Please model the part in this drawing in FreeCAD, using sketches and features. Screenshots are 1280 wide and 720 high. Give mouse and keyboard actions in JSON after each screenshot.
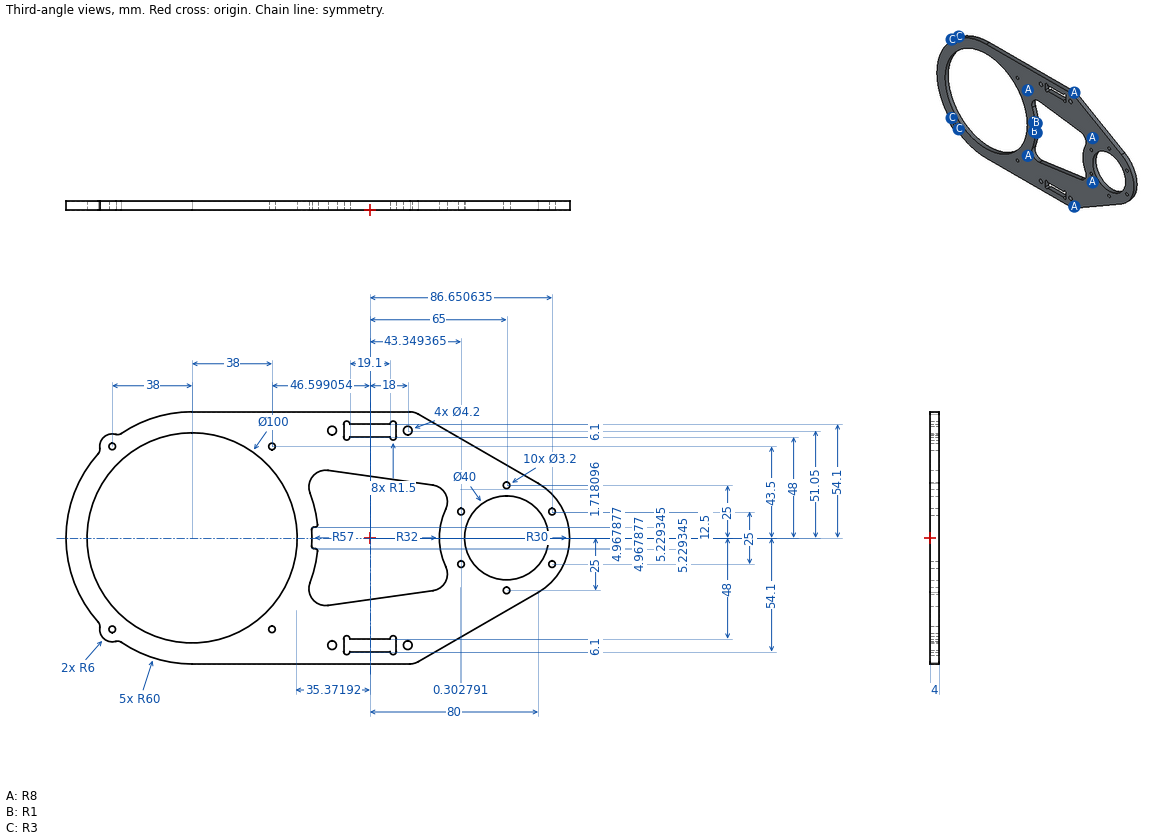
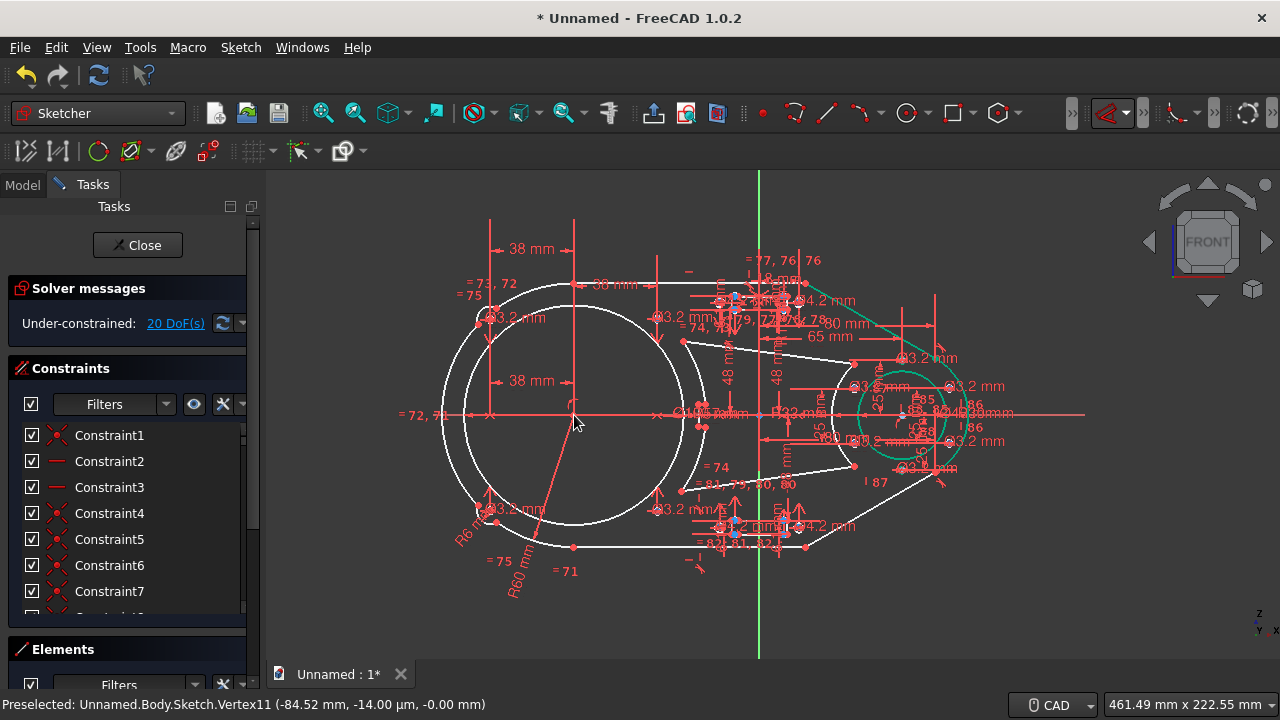
{"action": "left_click", "coordinate": [574, 547]}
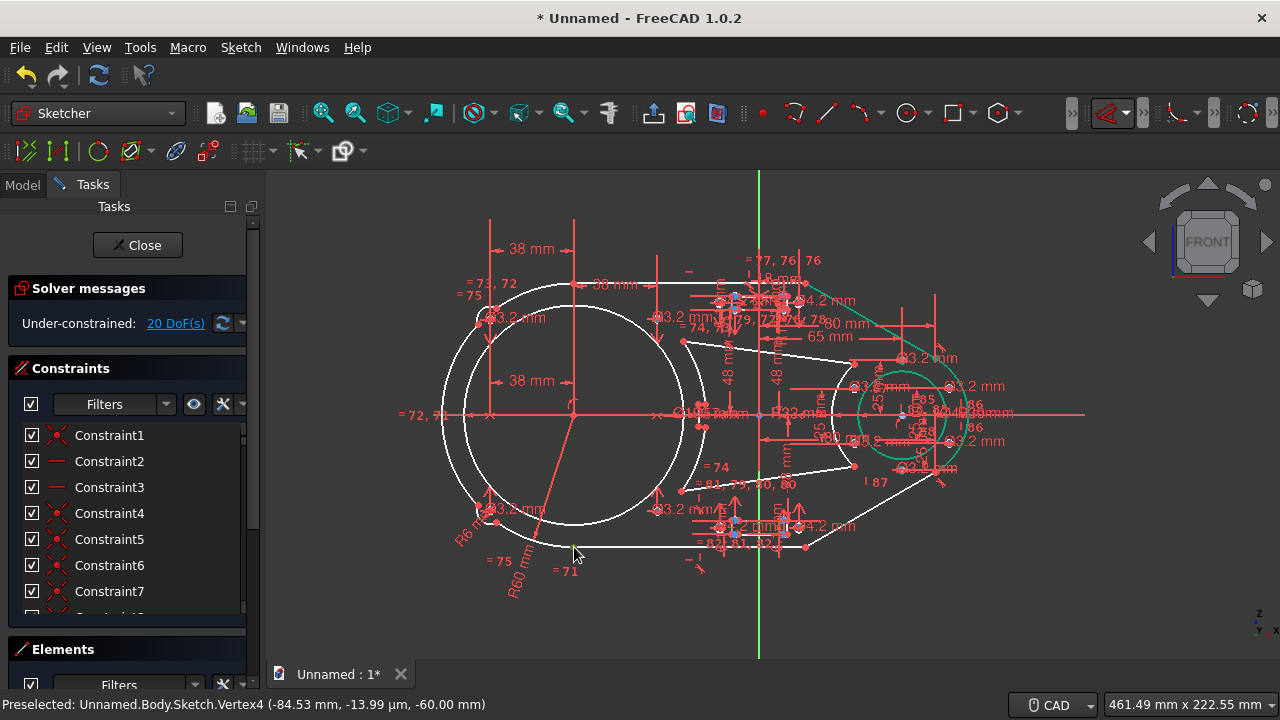
{"action": "left_click", "coordinate": [490, 511]}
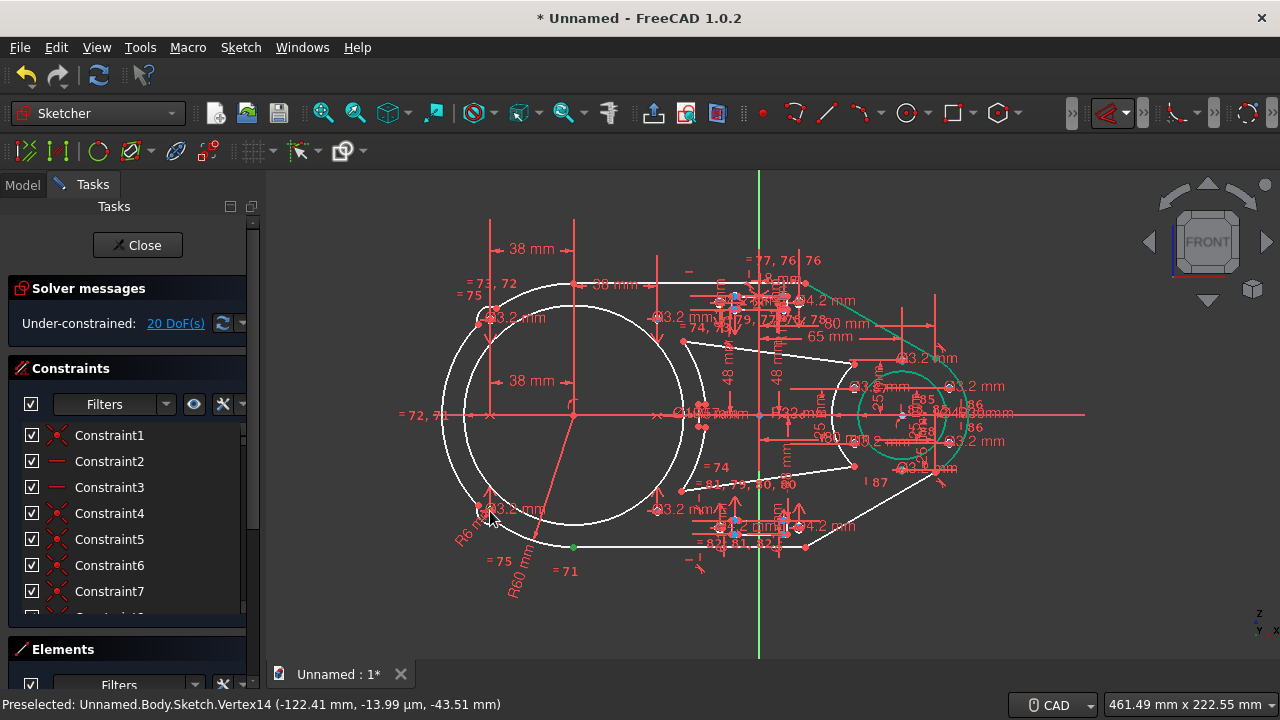
{"action": "left_click", "coordinate": [1128, 114]}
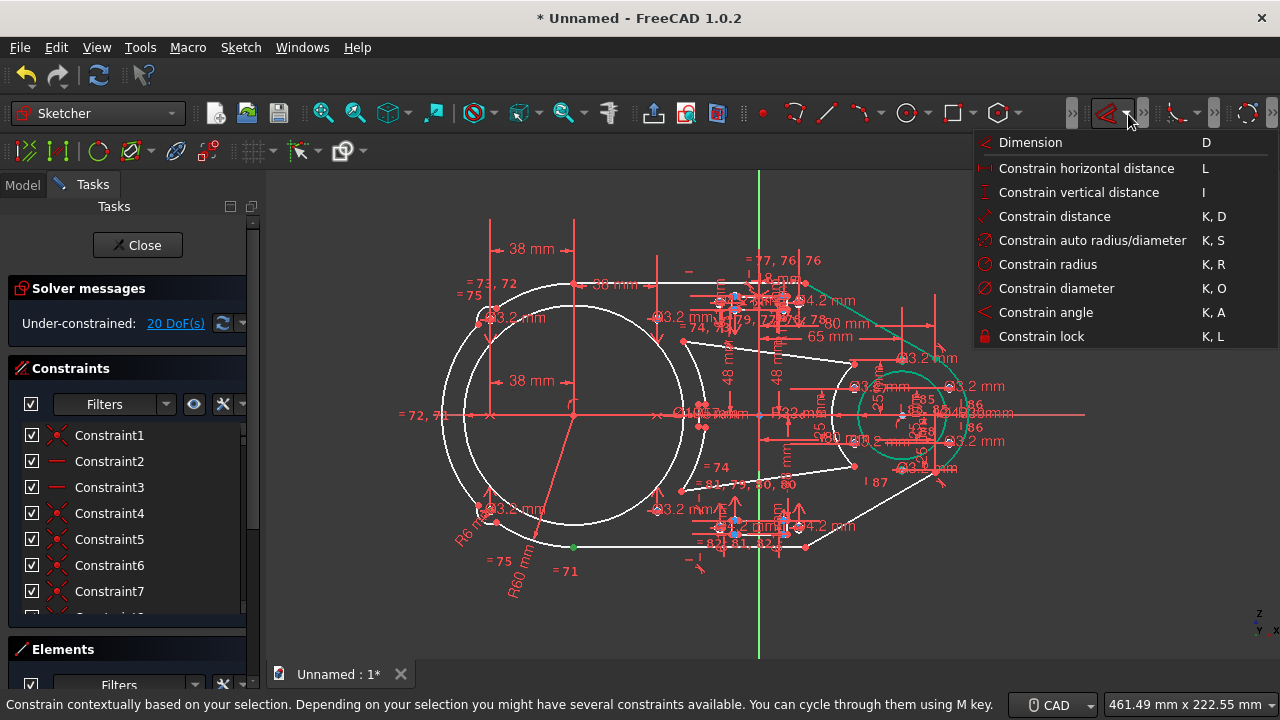
{"action": "left_click", "coordinate": [1126, 168]}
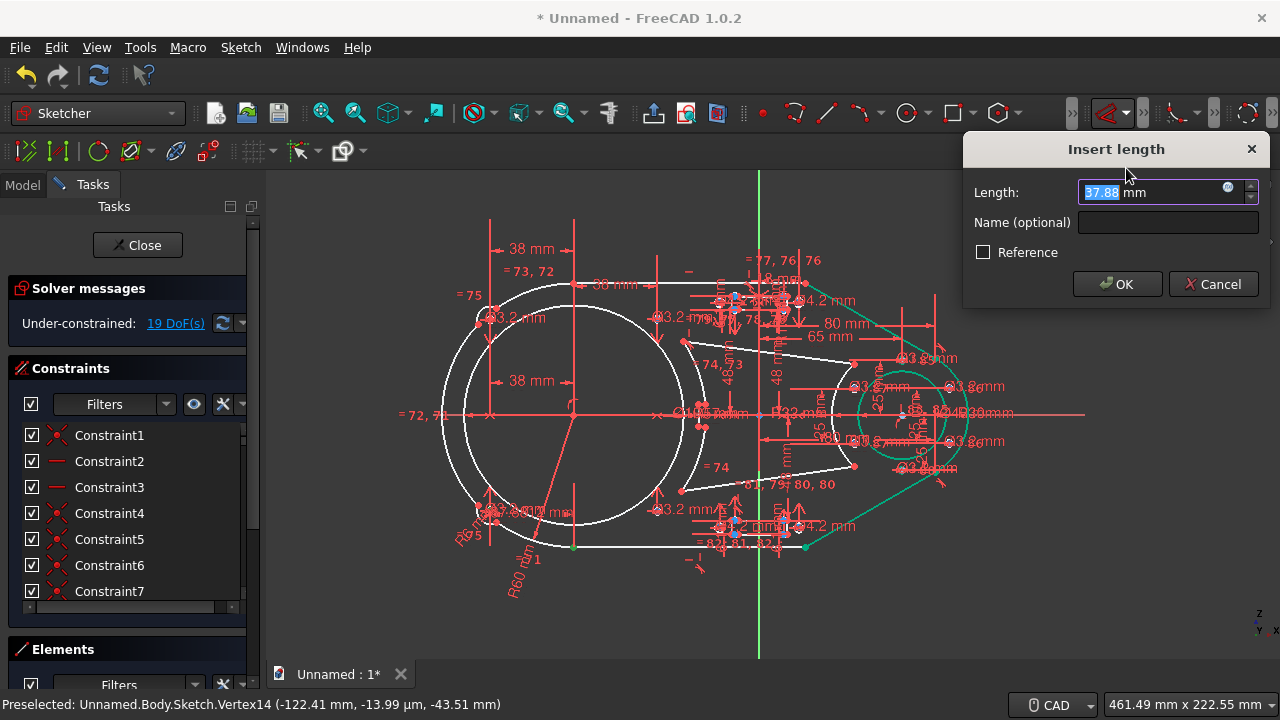
{"action": "type", "text": "38"}
{"action": "key", "text": "Return"}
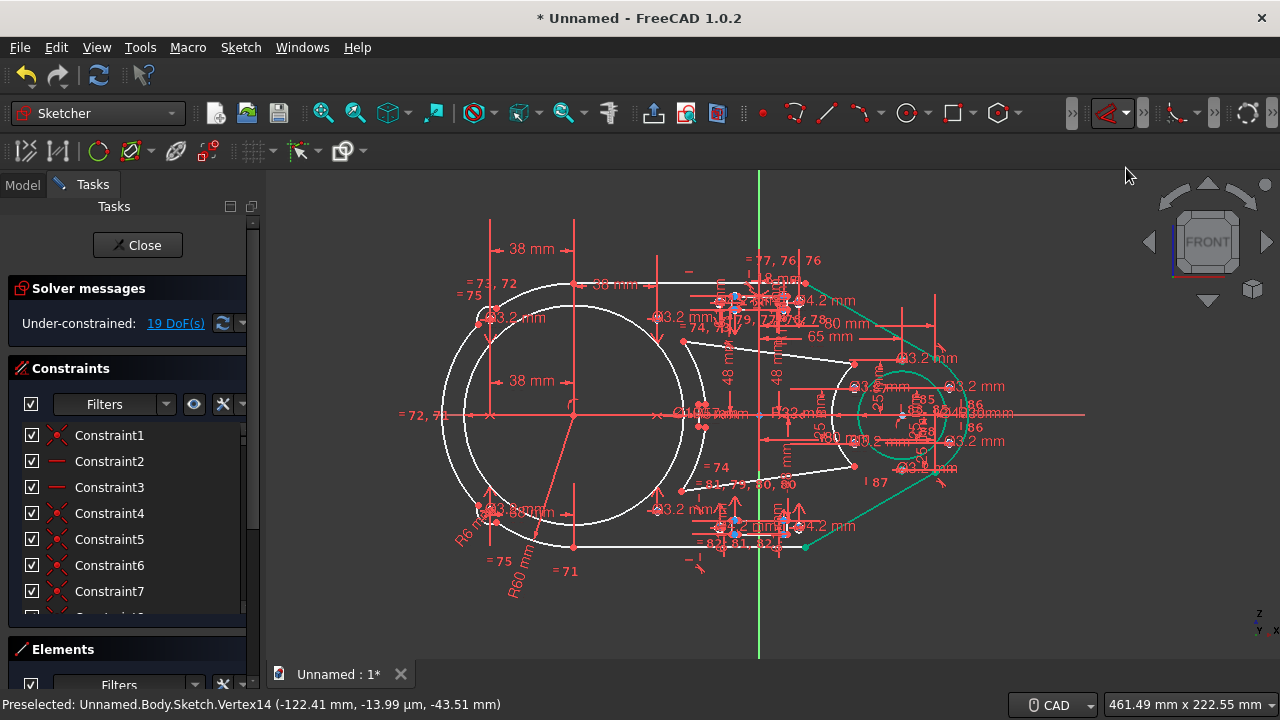
{"action": "left_click", "coordinate": [747, 310]}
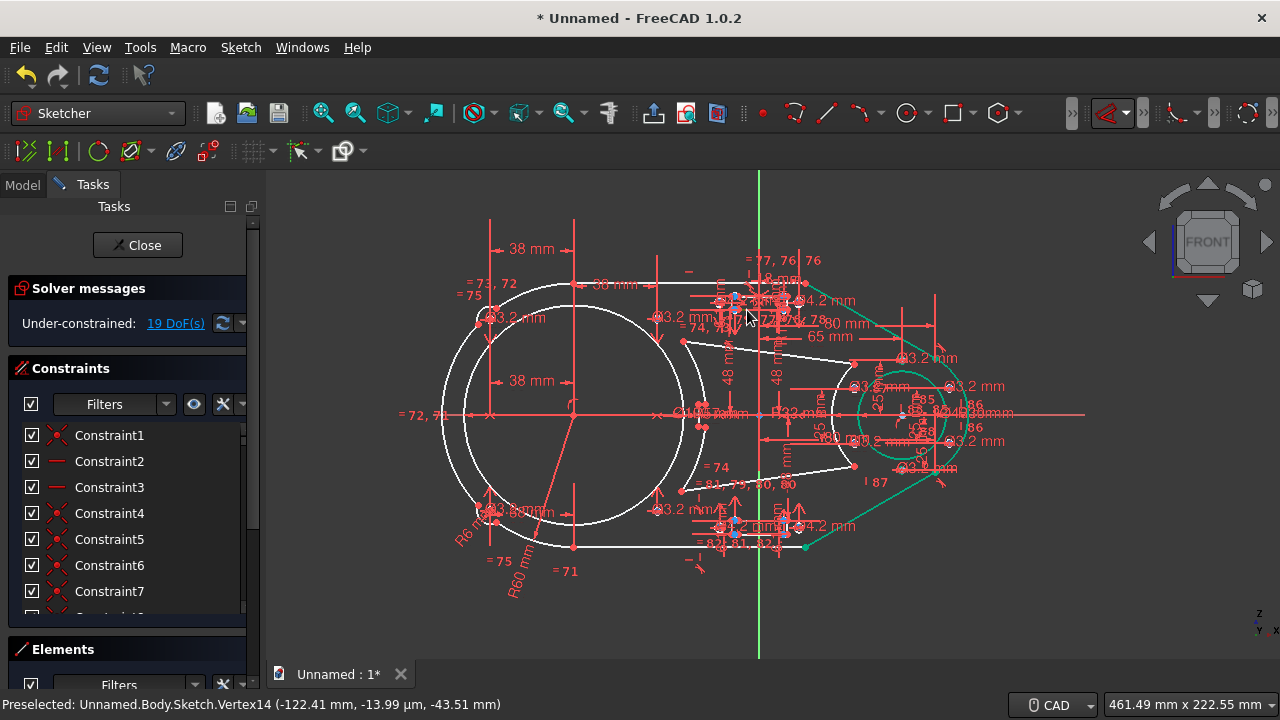
{"action": "key", "text": "l"}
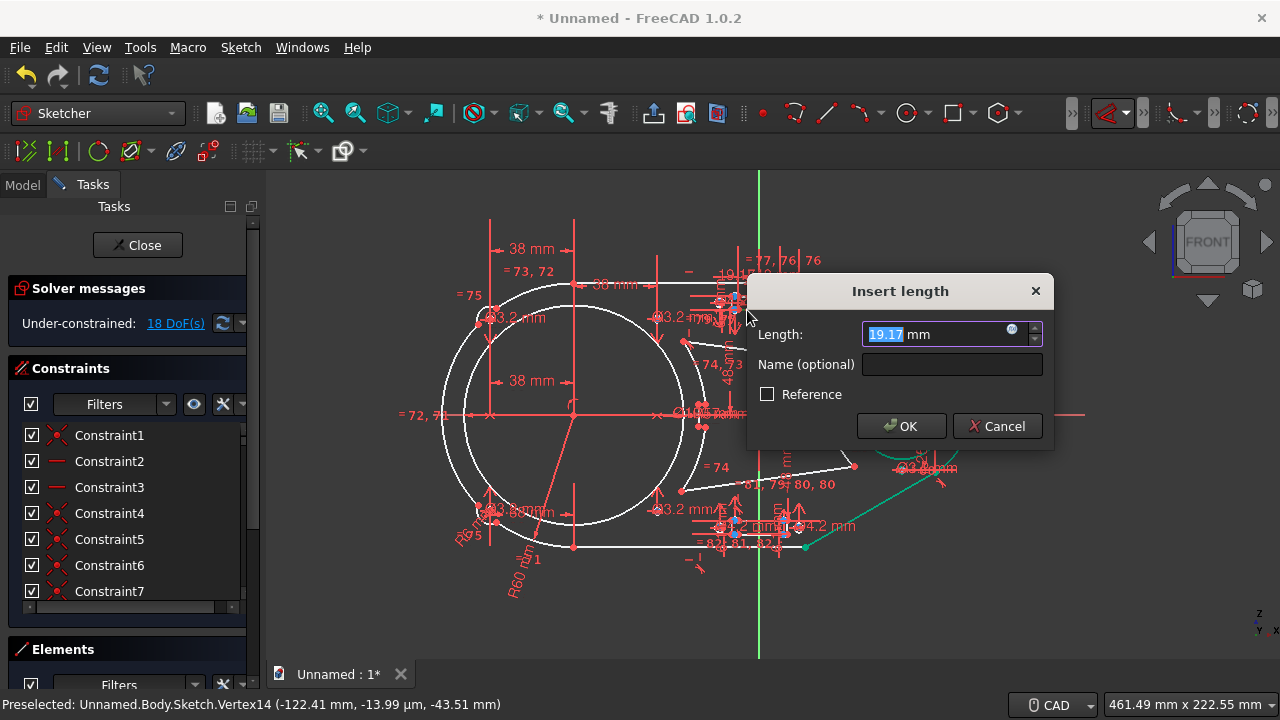
{"action": "type", "text": "19.1"}
{"action": "key", "text": "Return"}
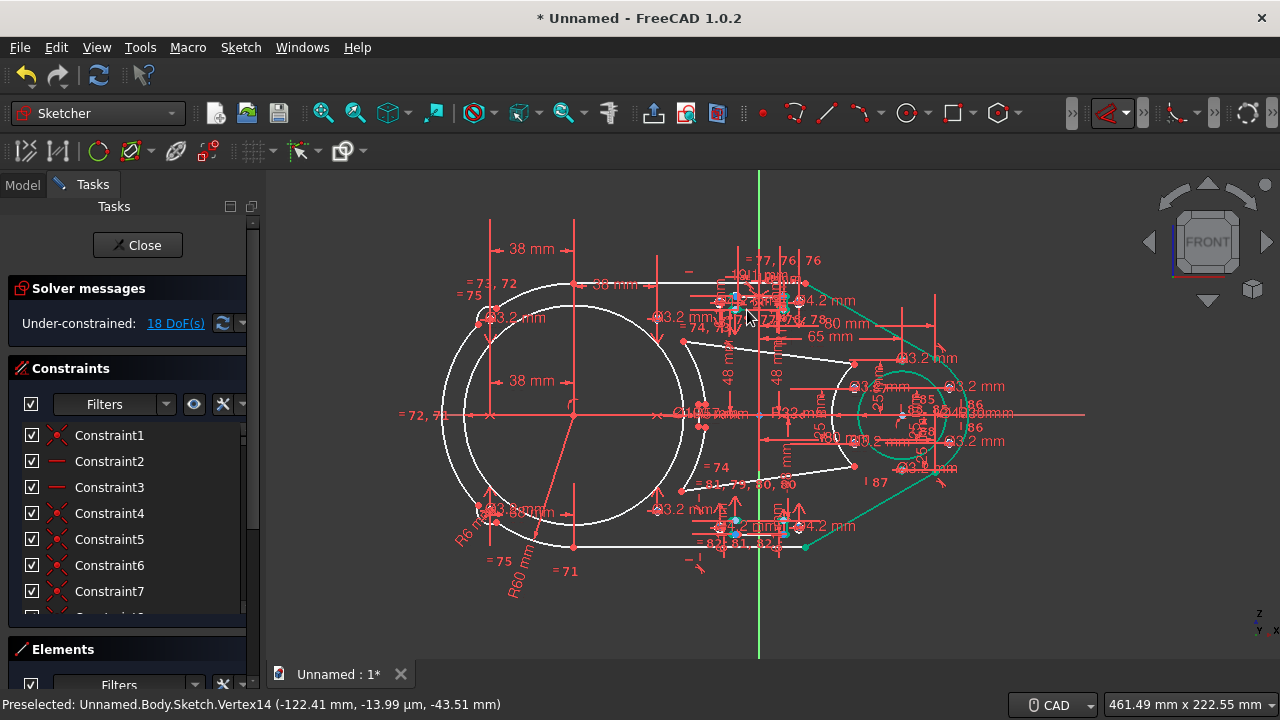
{"action": "scroll", "coordinate": [950, 388], "scroll_direction": "up", "scroll_amount": 2}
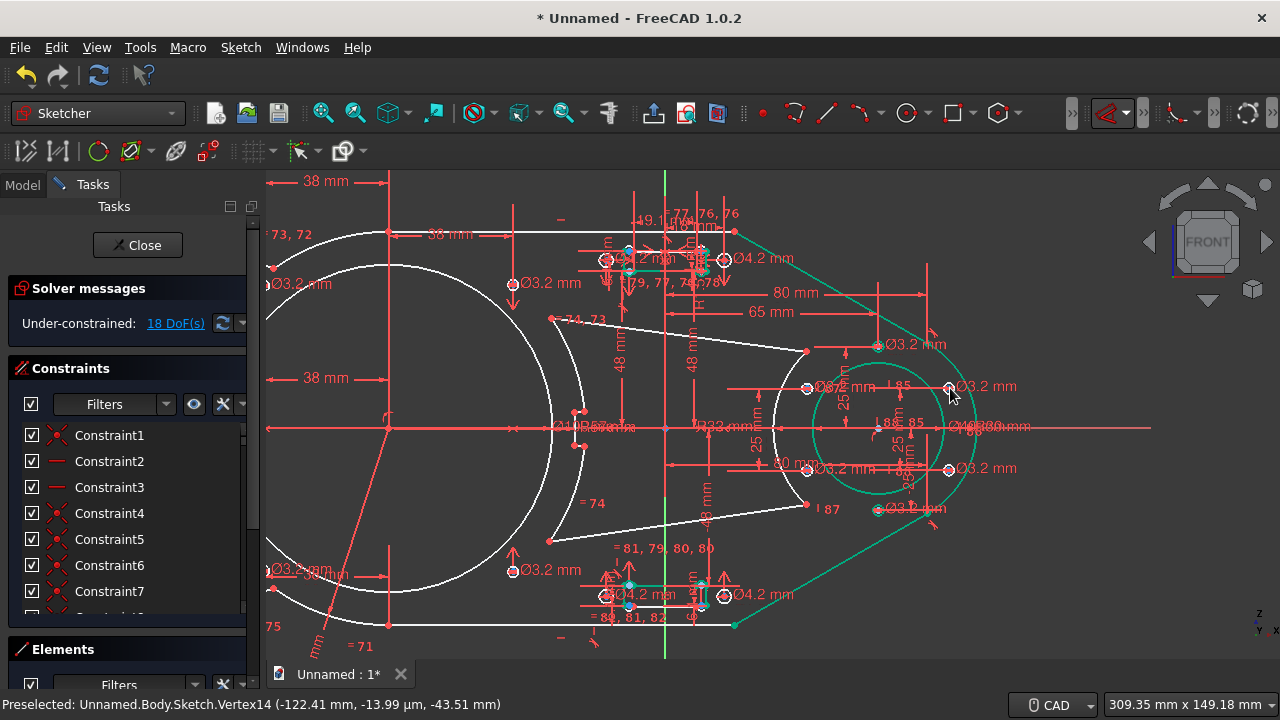
{"action": "left_click", "coordinate": [949, 388]}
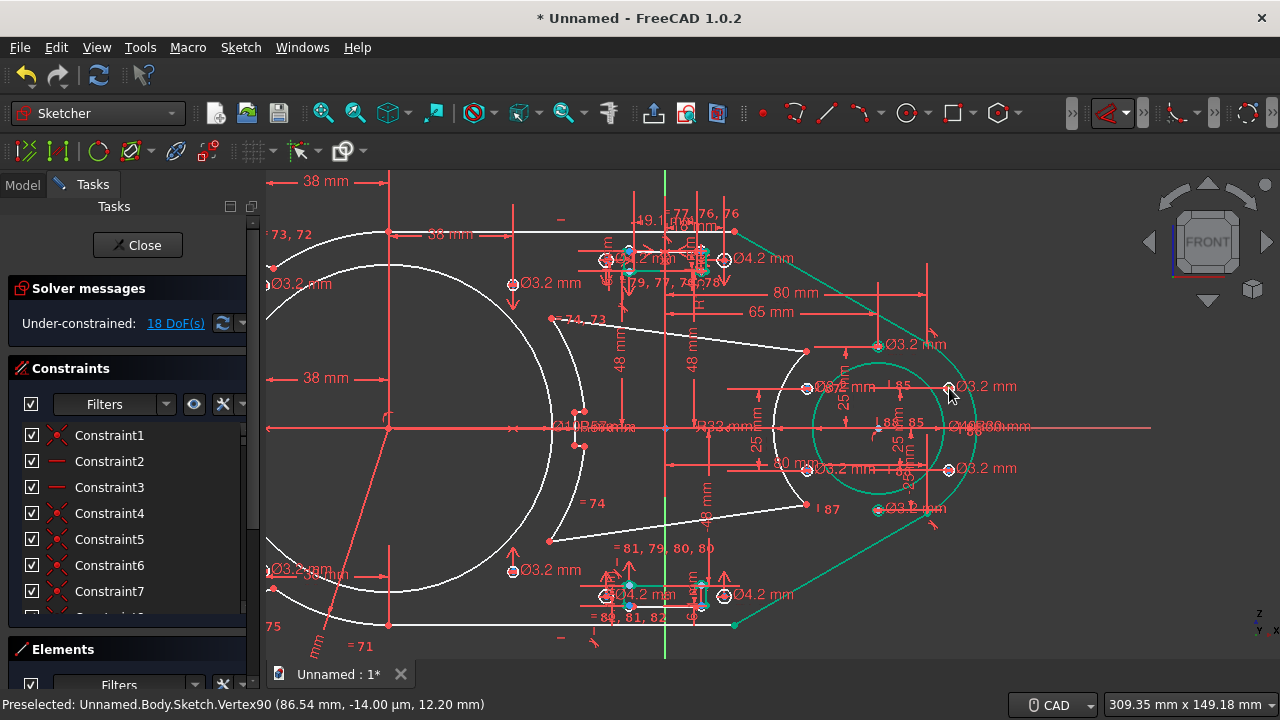
{"action": "left_click", "coordinate": [1128, 114]}